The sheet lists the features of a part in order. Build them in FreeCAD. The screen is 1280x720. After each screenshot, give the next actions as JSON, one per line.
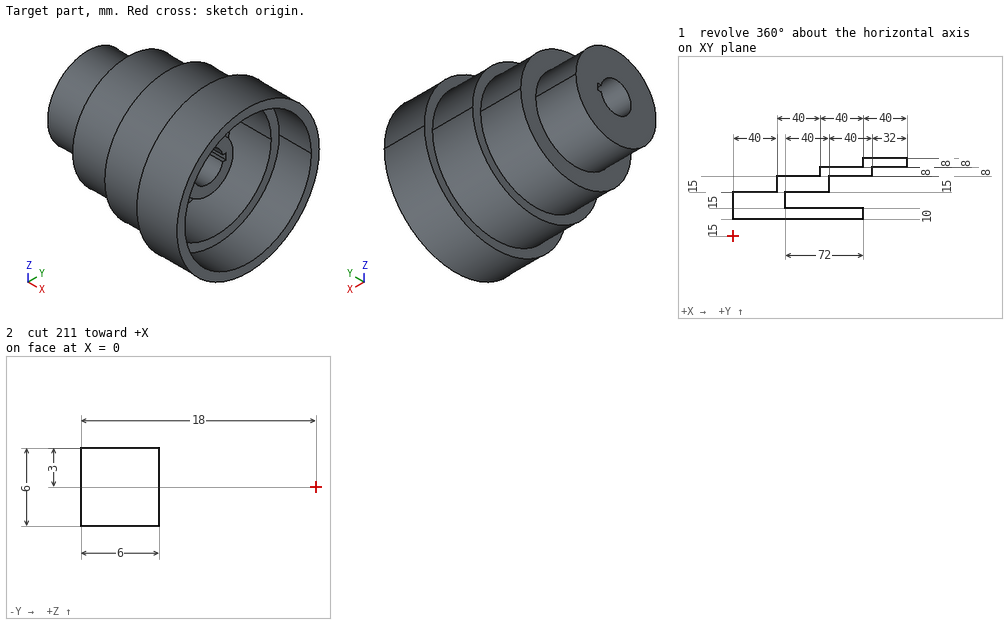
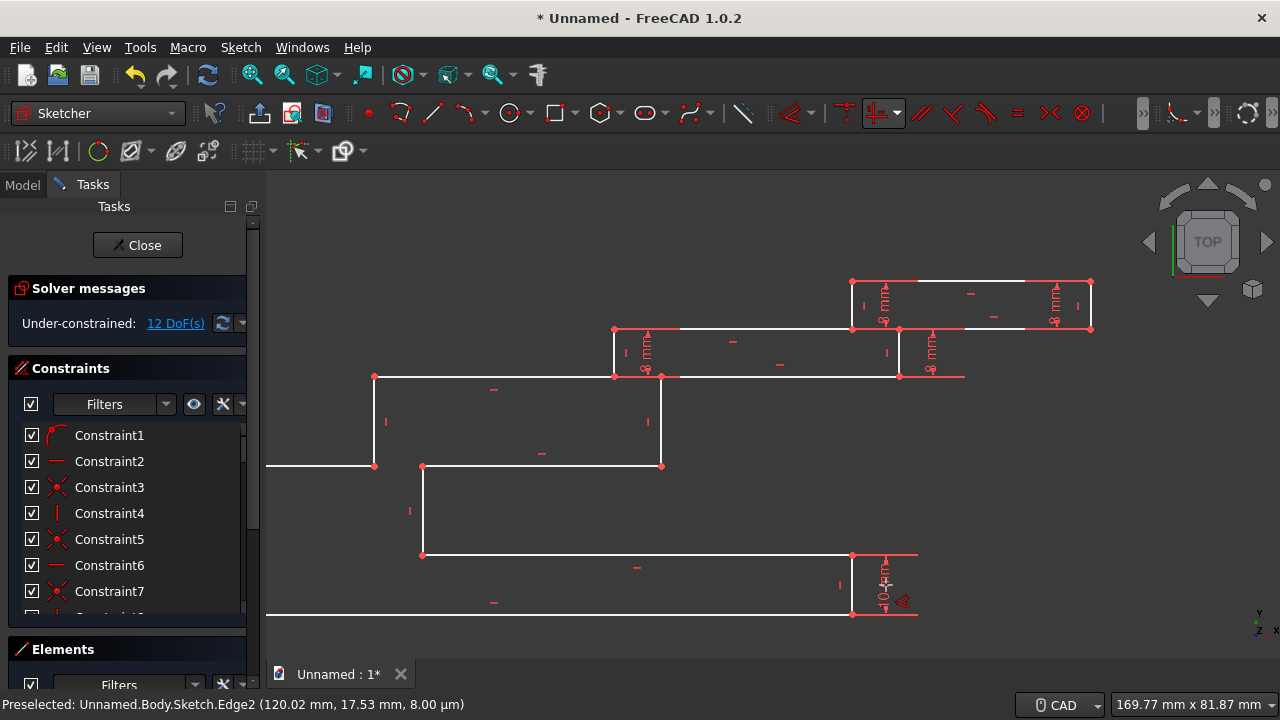
{"action": "left_click", "coordinate": [724, 555]}
{"action": "left_click", "coordinate": [638, 589]}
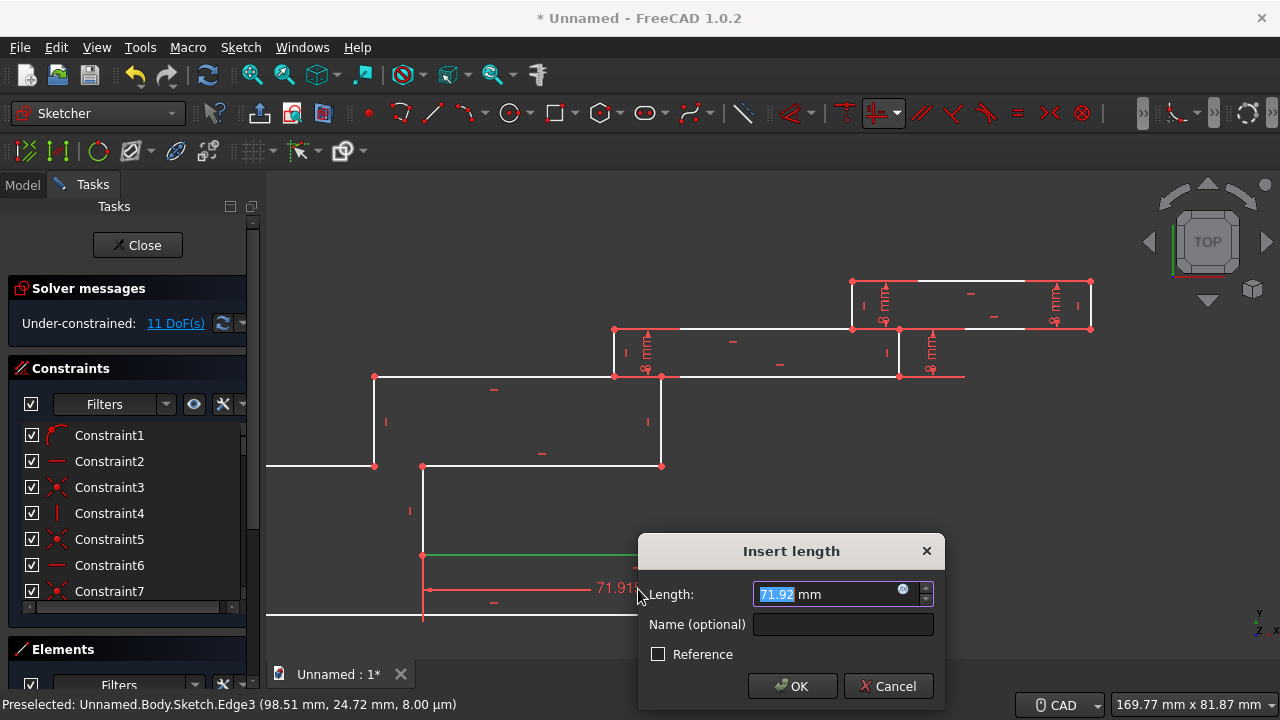
{"action": "type", "text": "72"}
{"action": "key", "text": "Return"}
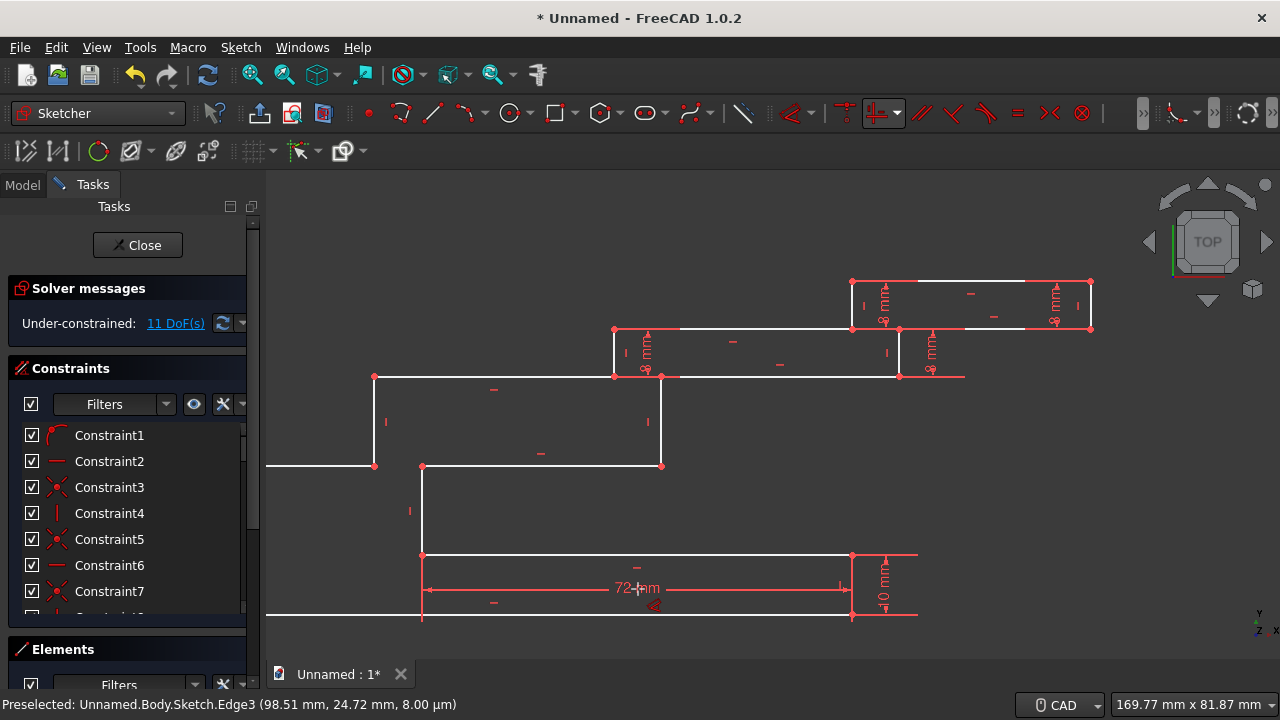
{"action": "left_click", "coordinate": [422, 528]}
{"action": "left_click", "coordinate": [388, 511]}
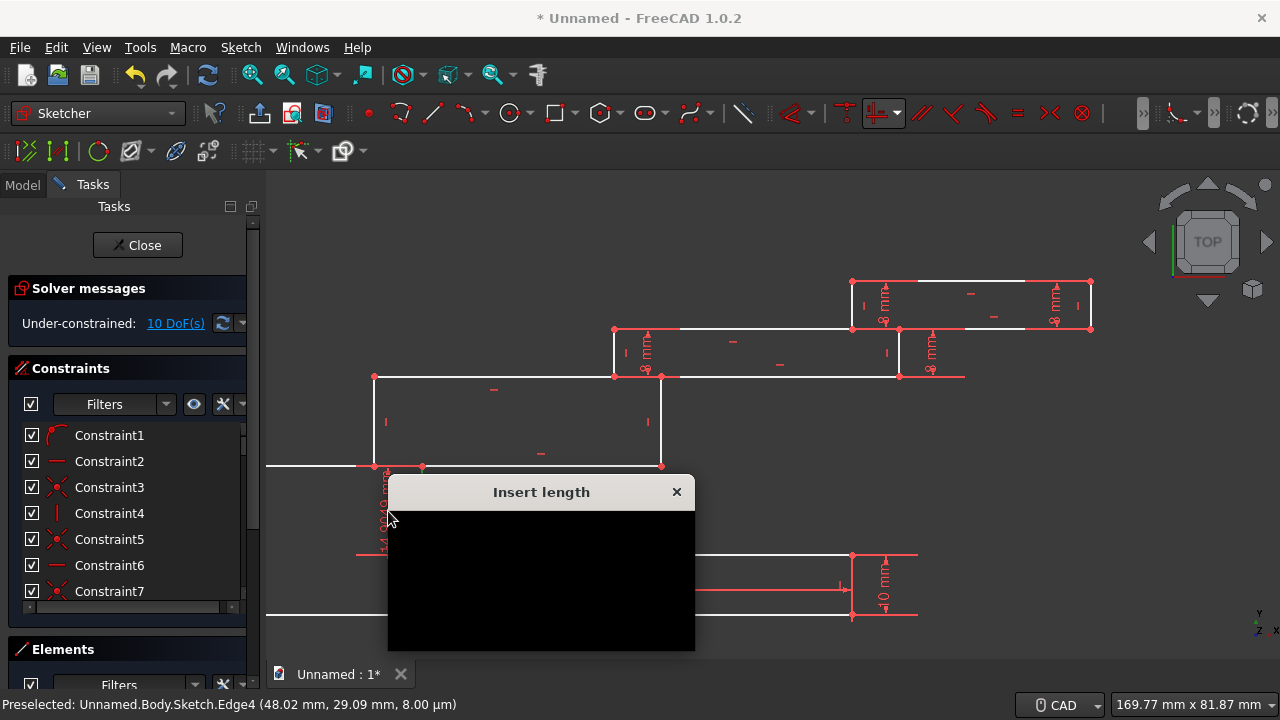
{"action": "type", "text": "15"}
{"action": "key", "text": "Return"}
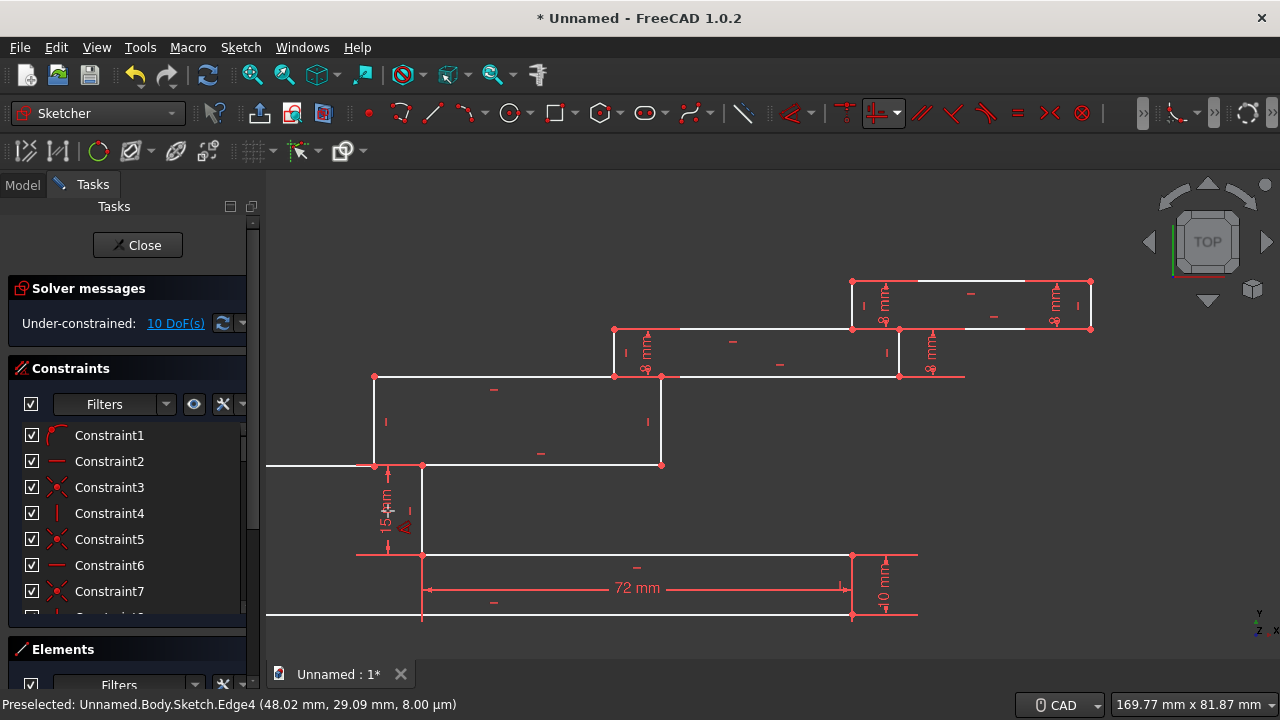
{"action": "left_click", "coordinate": [494, 465]}
{"action": "left_click", "coordinate": [542, 431]}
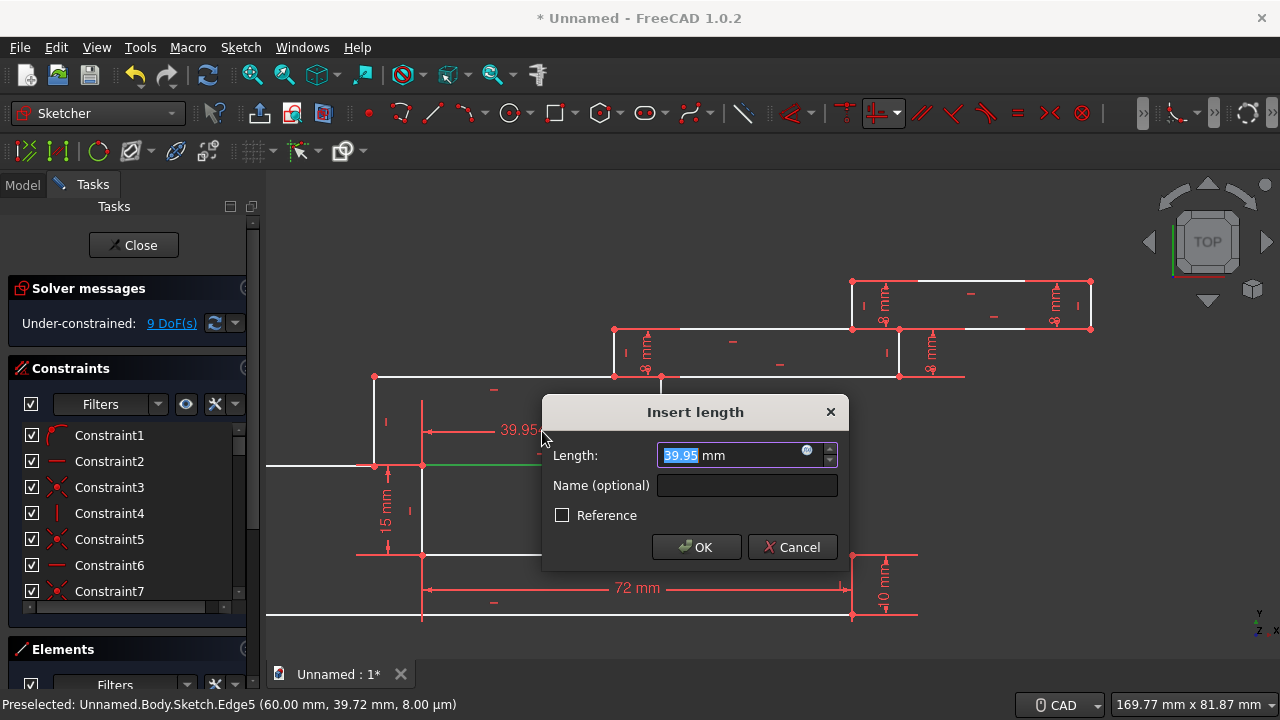
{"action": "type", "text": "40"}
{"action": "key", "text": "Return"}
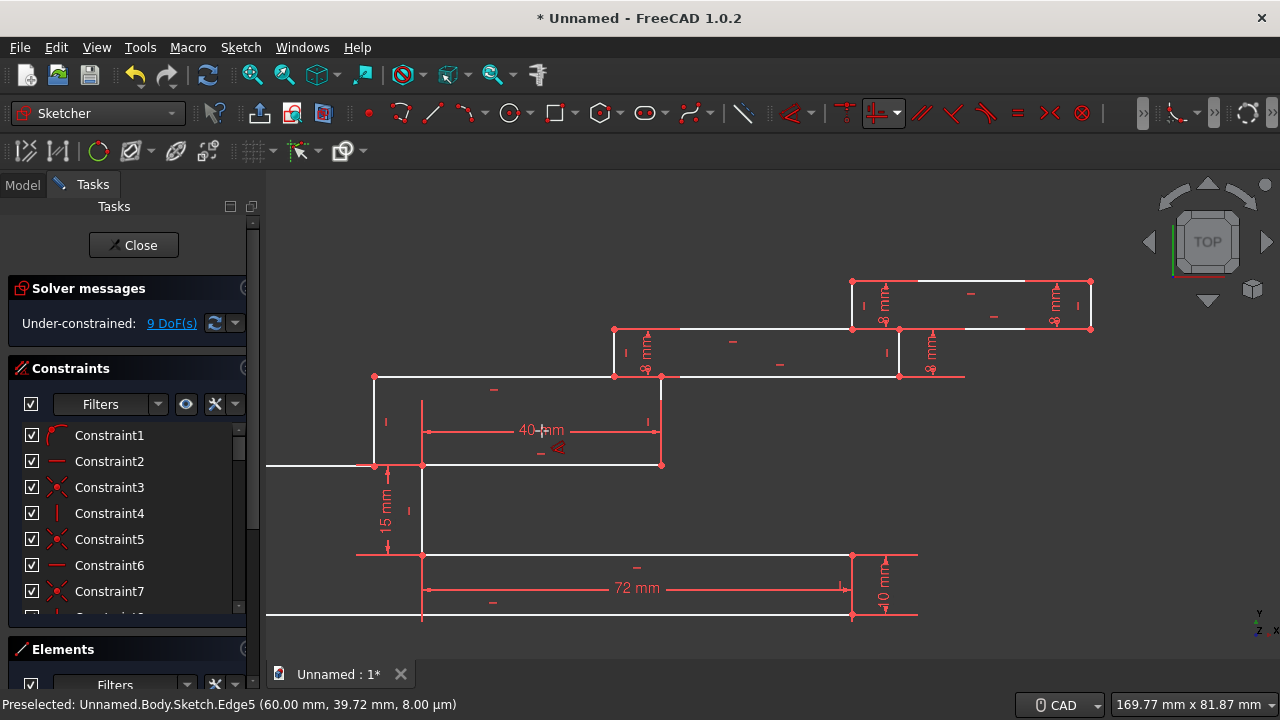
{"action": "left_click", "coordinate": [661, 439]}
{"action": "left_click", "coordinate": [695, 421]}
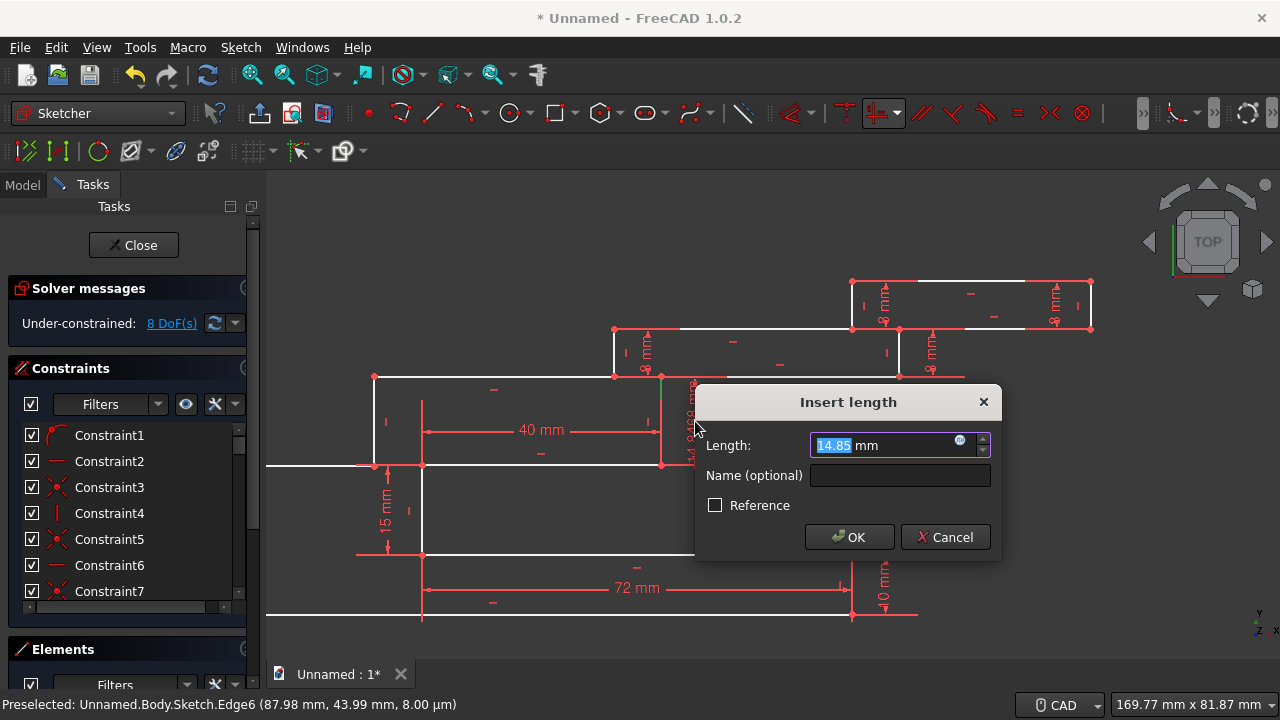
{"action": "type", "text": "15"}
{"action": "key", "text": "Return"}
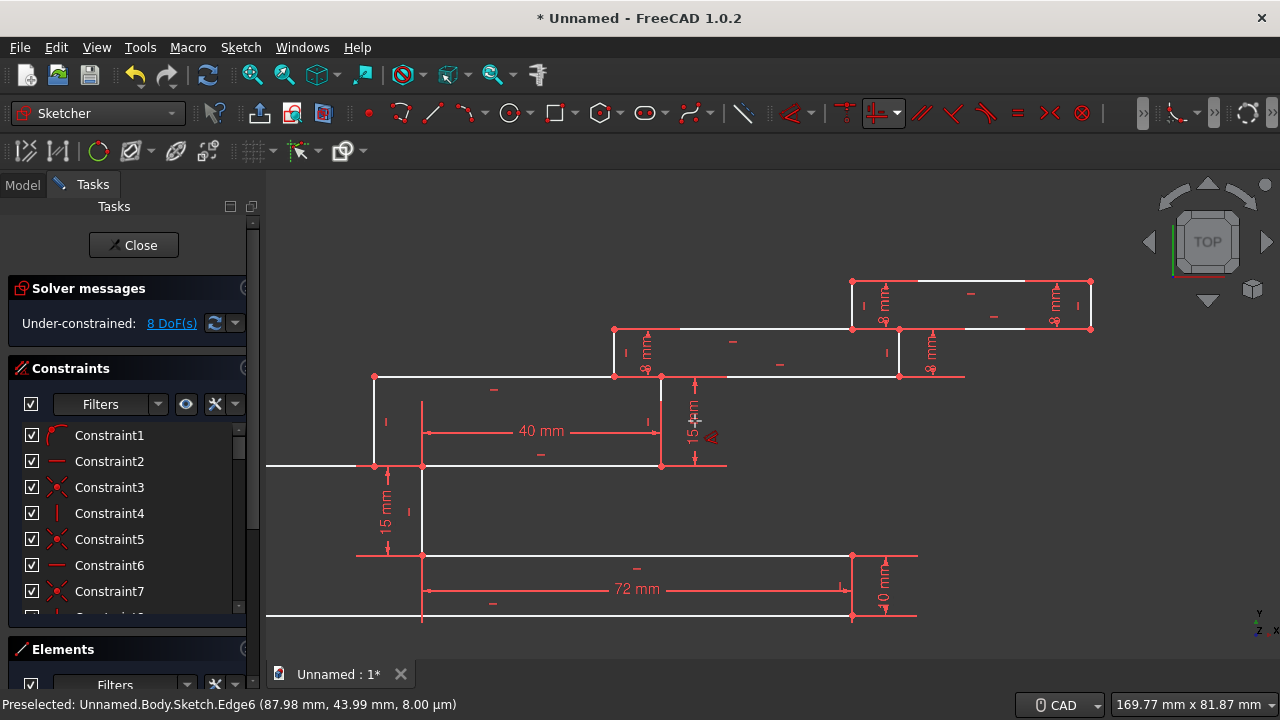
{"action": "left_click", "coordinate": [733, 377]}
{"action": "left_click", "coordinate": [780, 343]}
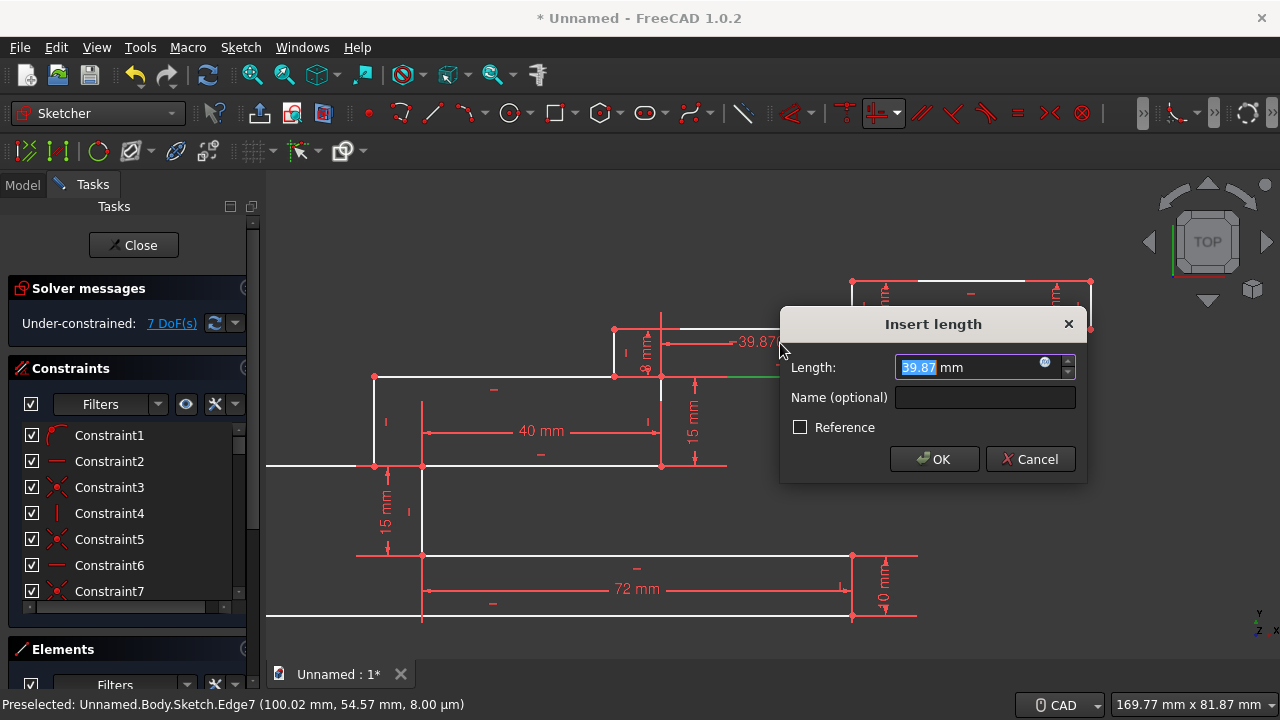
{"action": "type", "text": "40"}
{"action": "key", "text": "Return"}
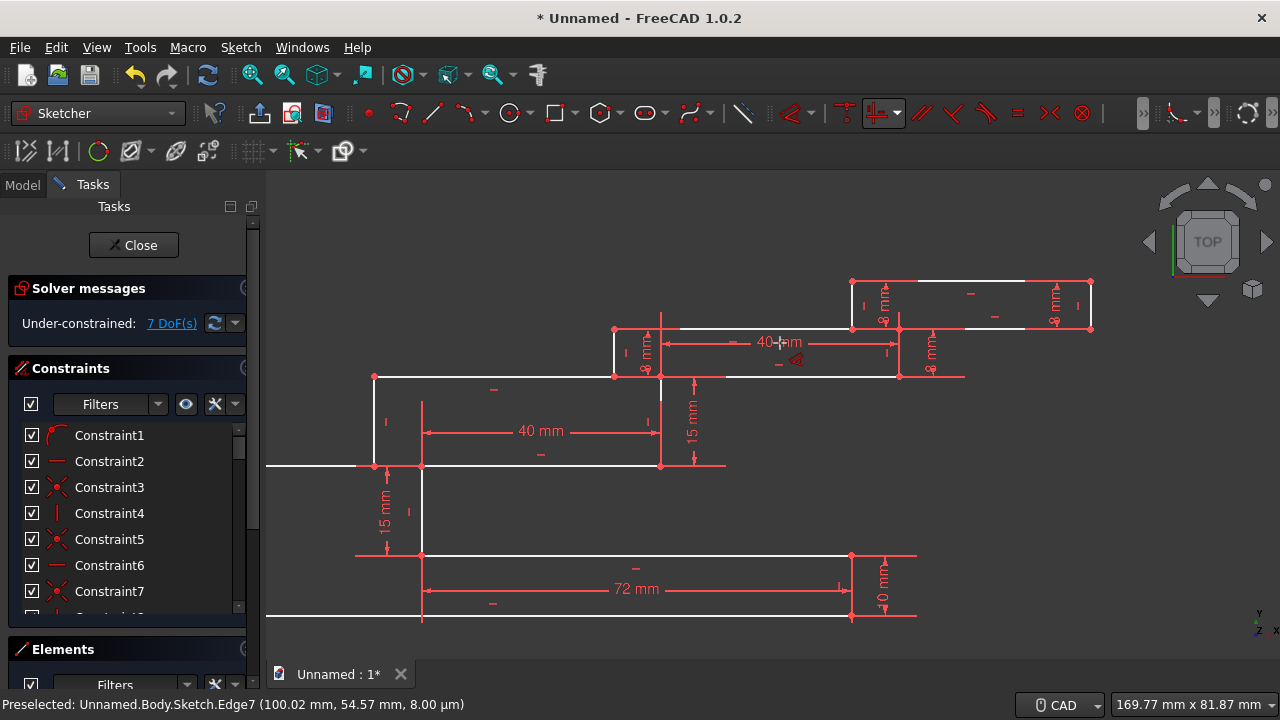
{"action": "left_click", "coordinate": [957, 329]}
{"action": "left_click", "coordinate": [1039, 363]}